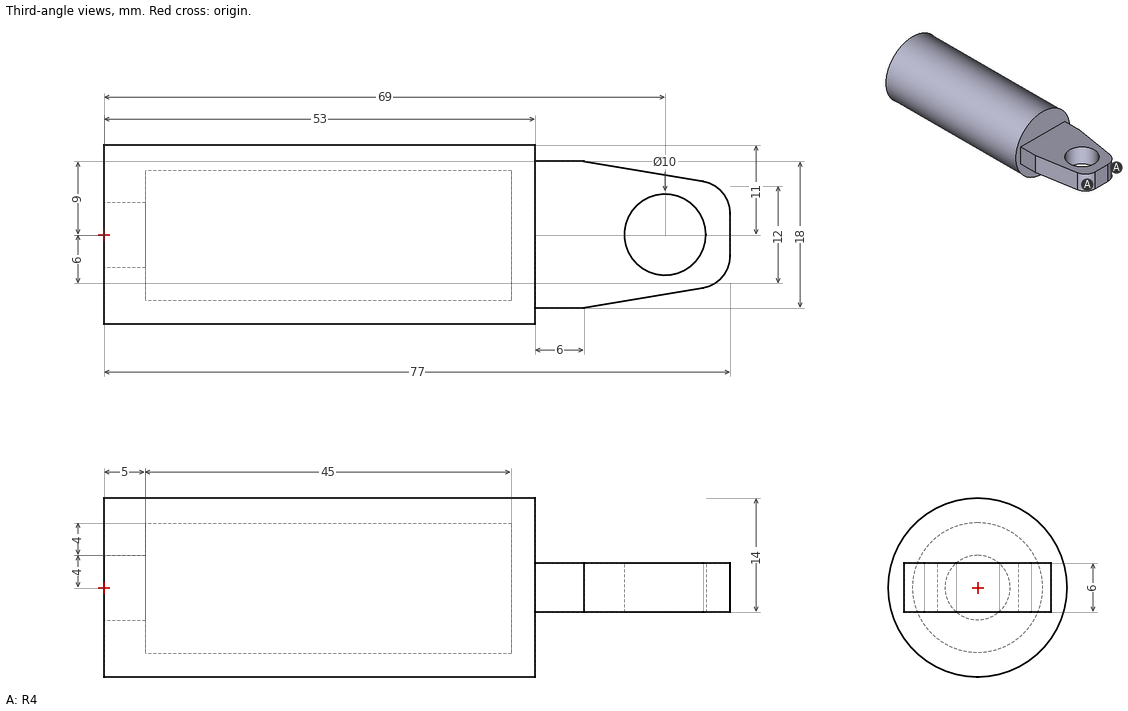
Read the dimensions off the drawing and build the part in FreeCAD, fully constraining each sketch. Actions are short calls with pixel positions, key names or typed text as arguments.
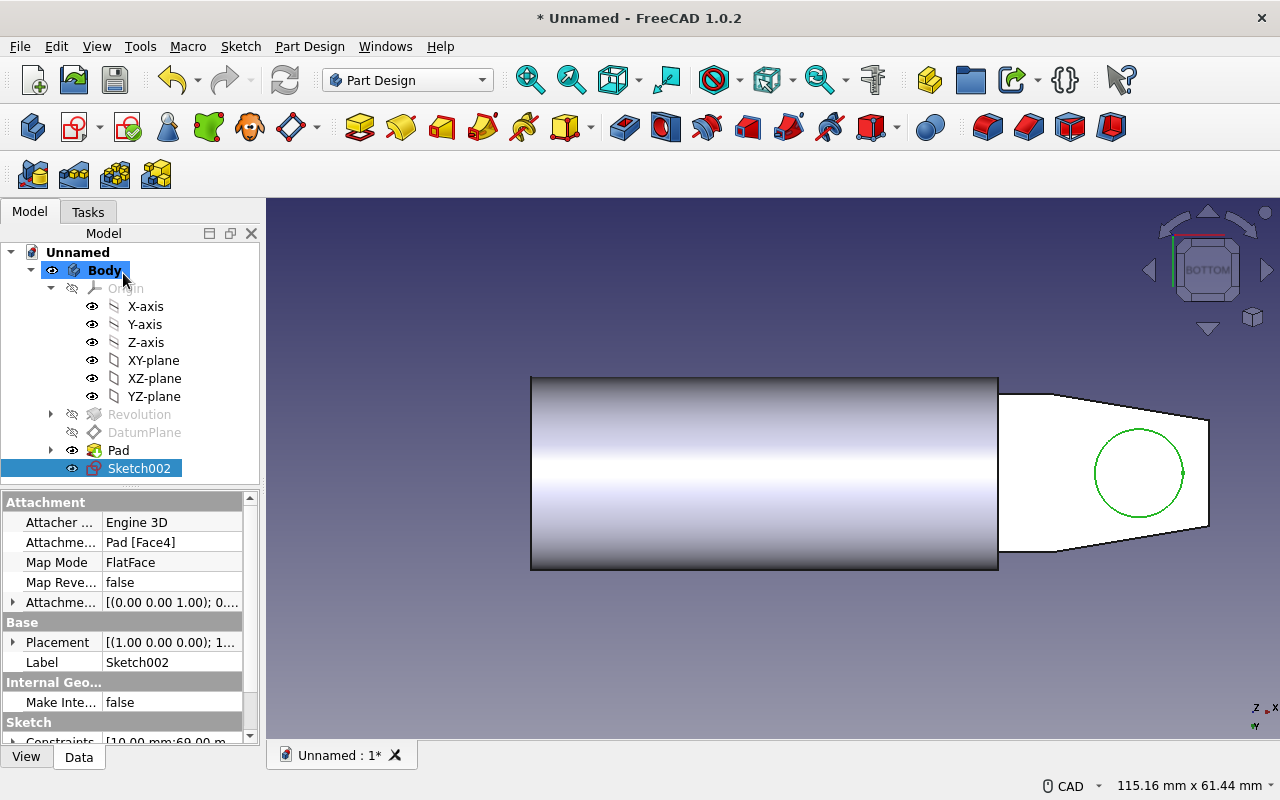
click(625, 128)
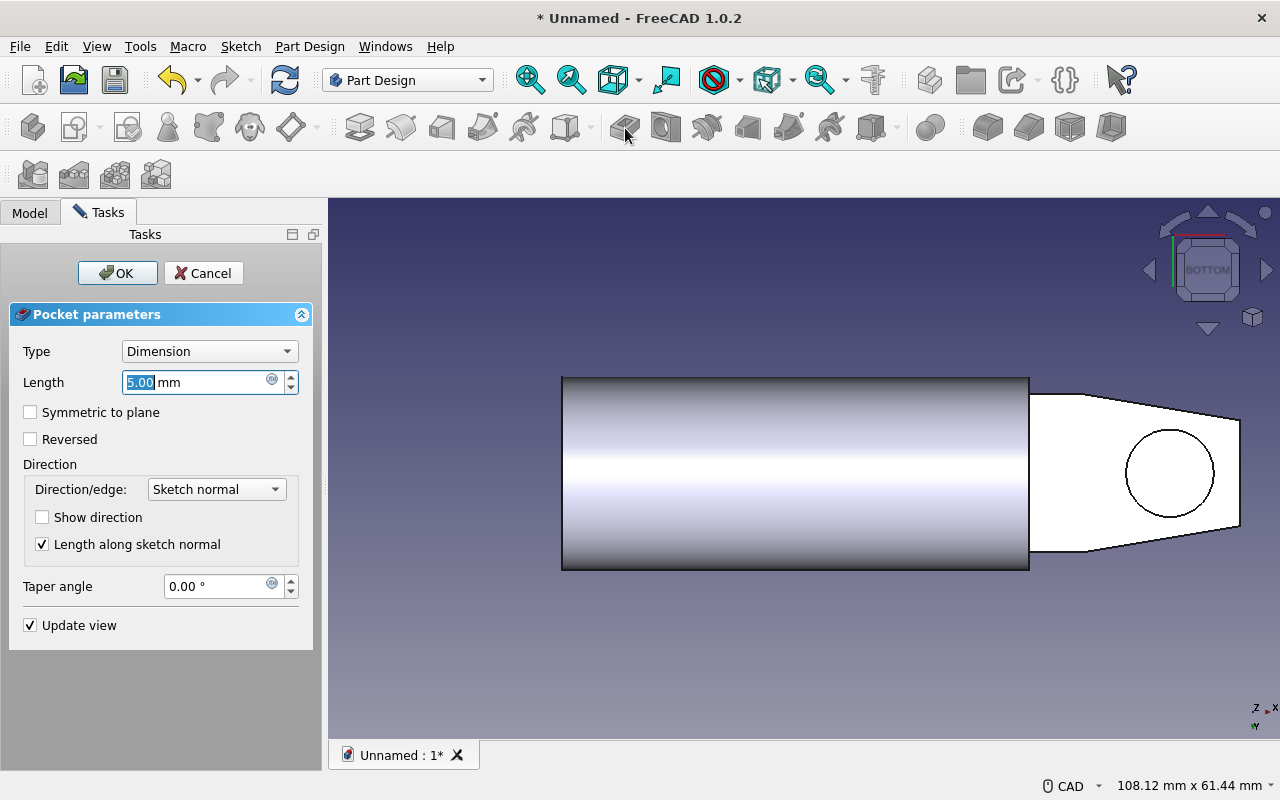
text(14)
key(Tab)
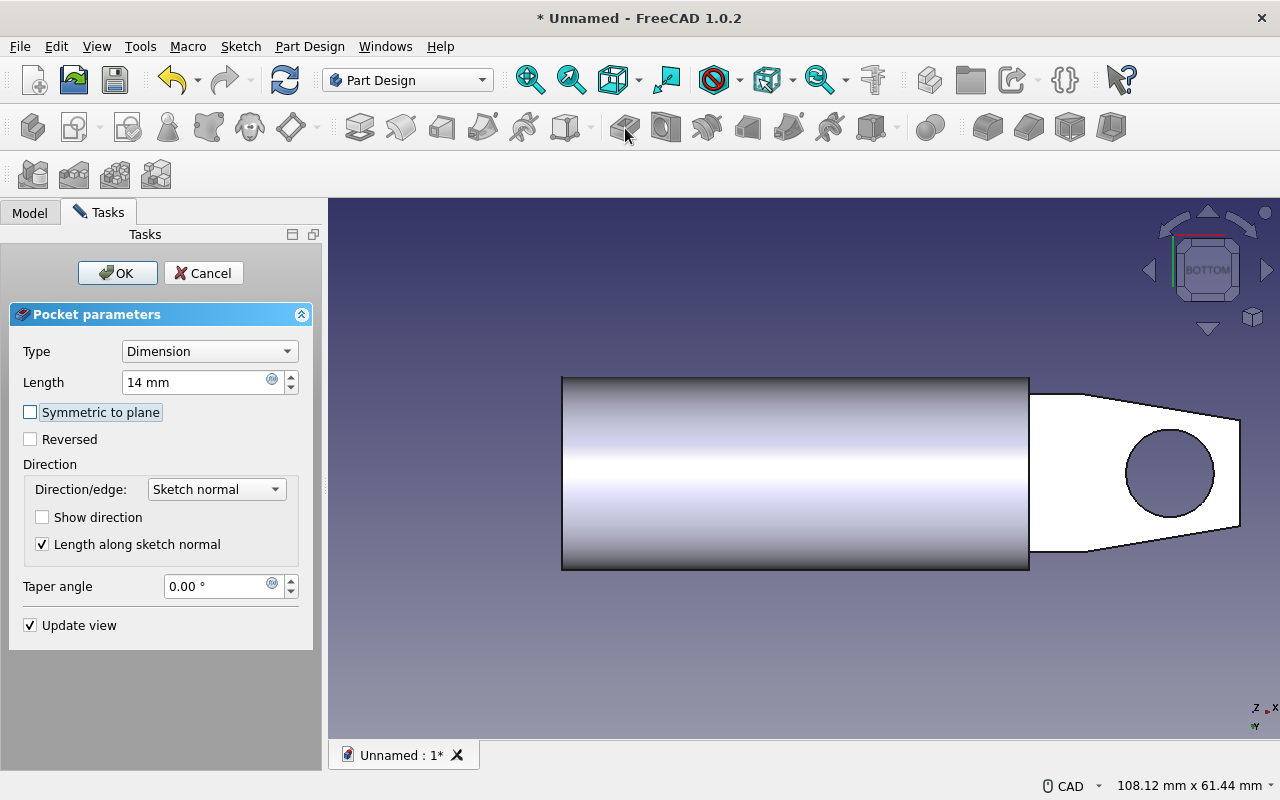
click(118, 273)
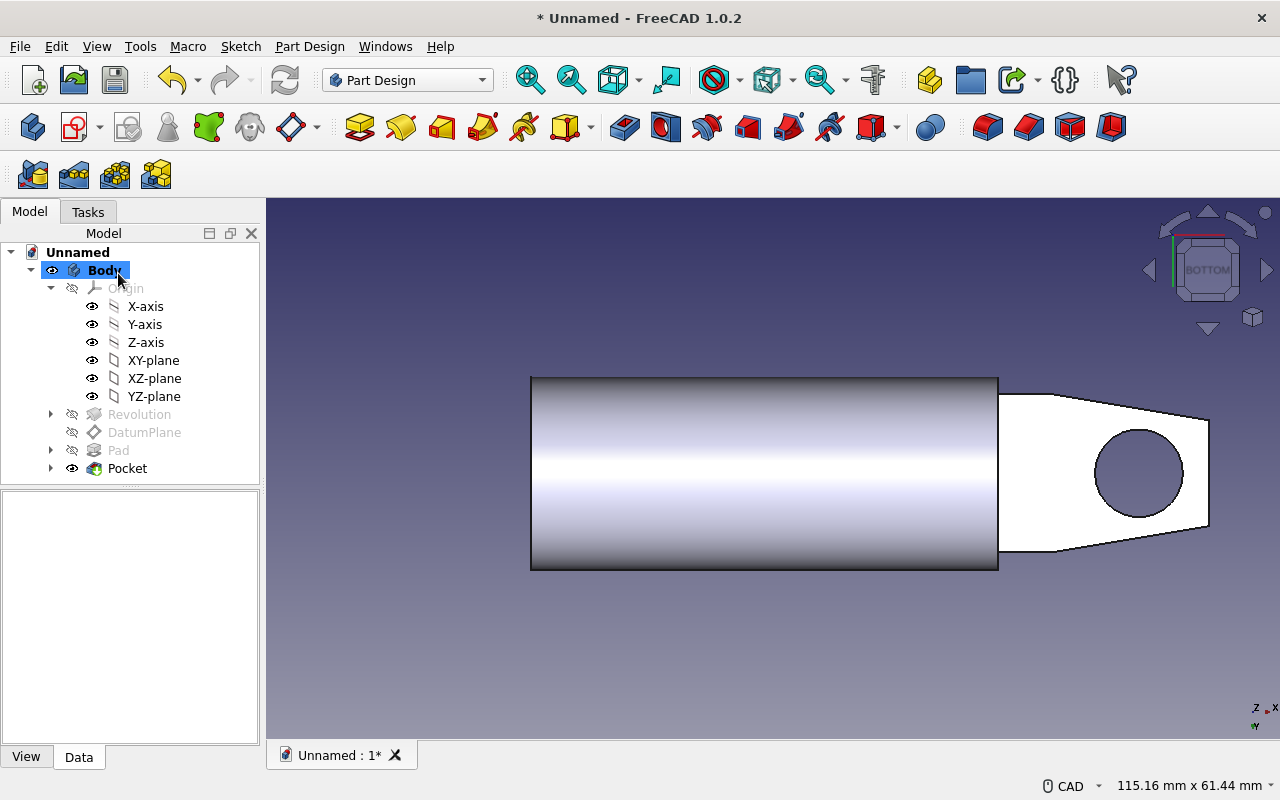
click(74, 128)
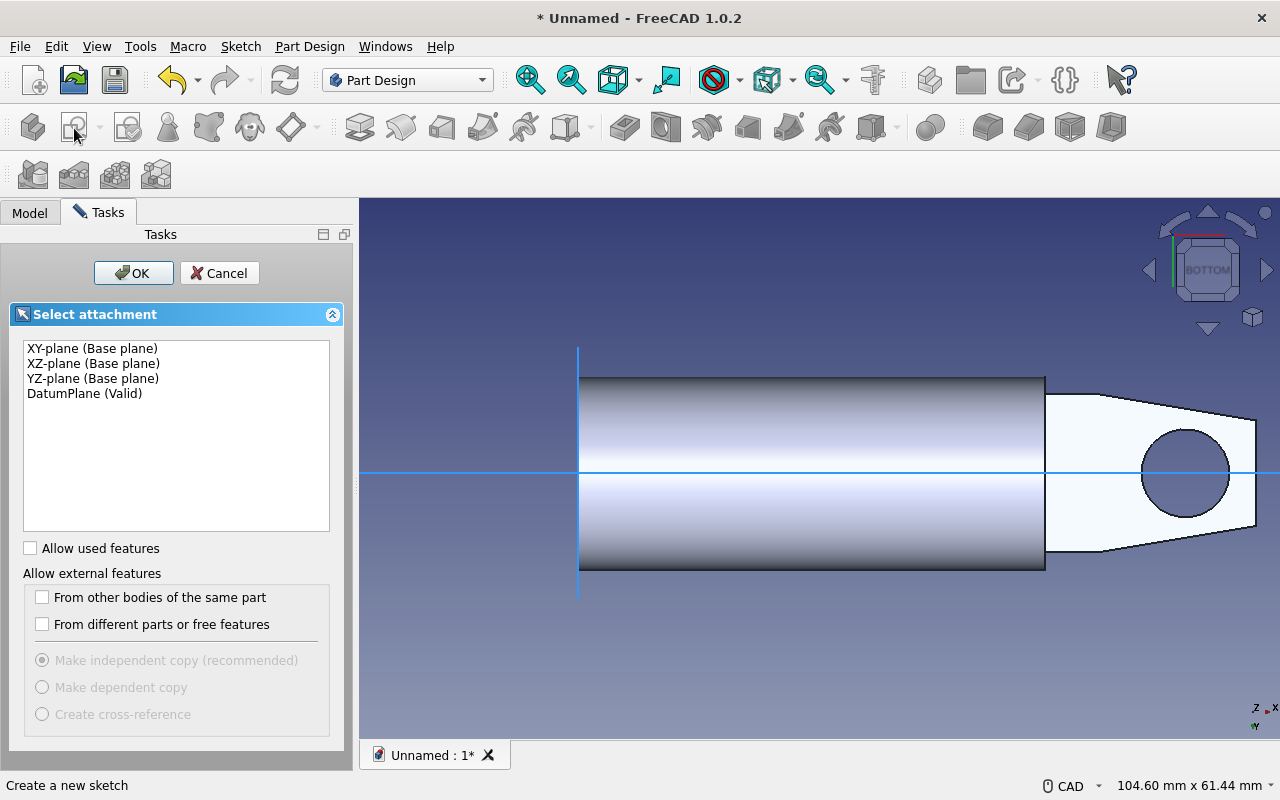
click(84, 364)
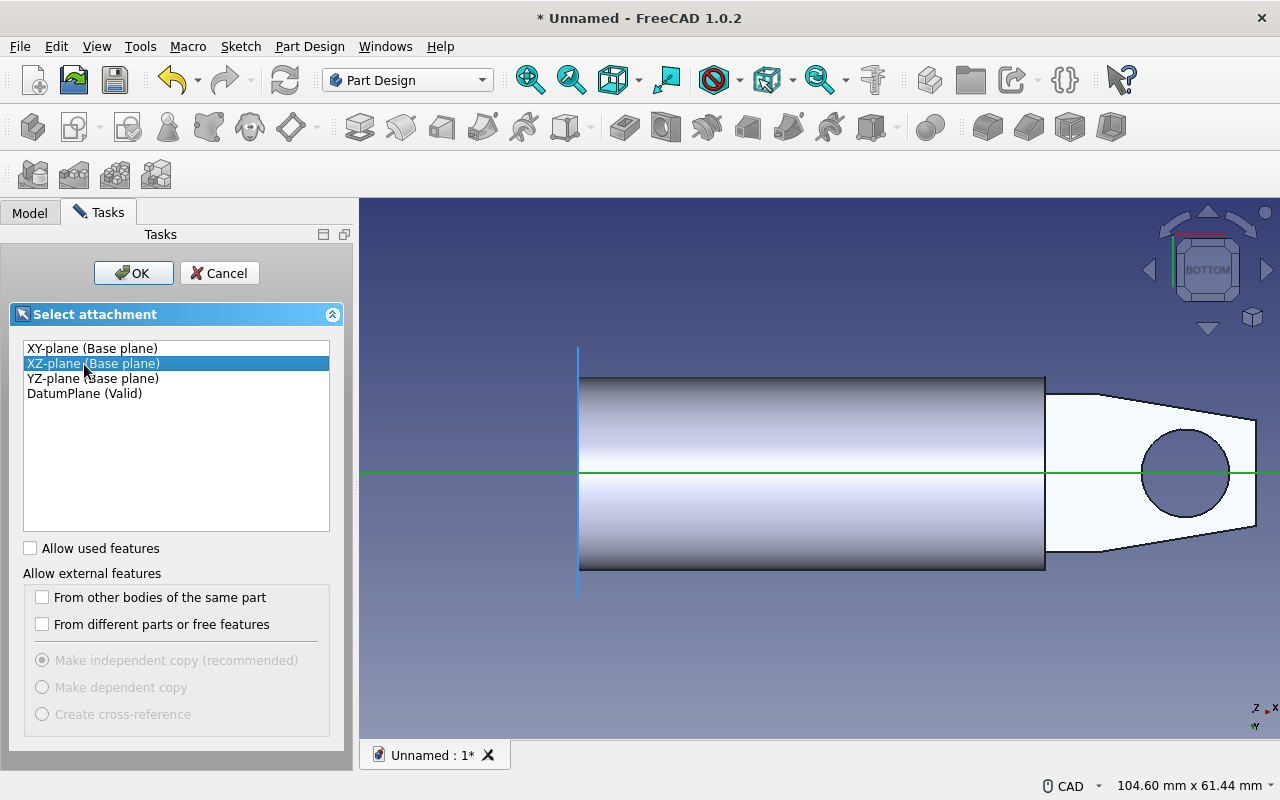
click(134, 273)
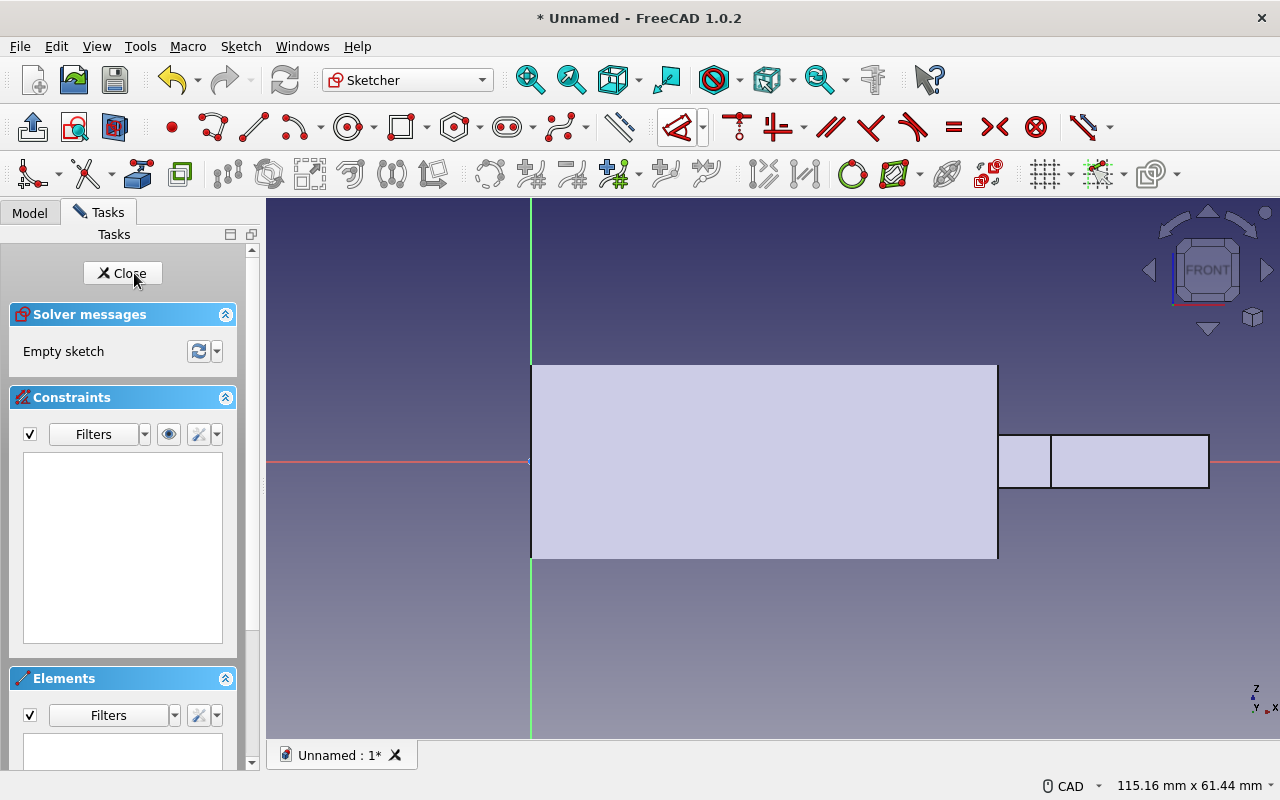
click(115, 128)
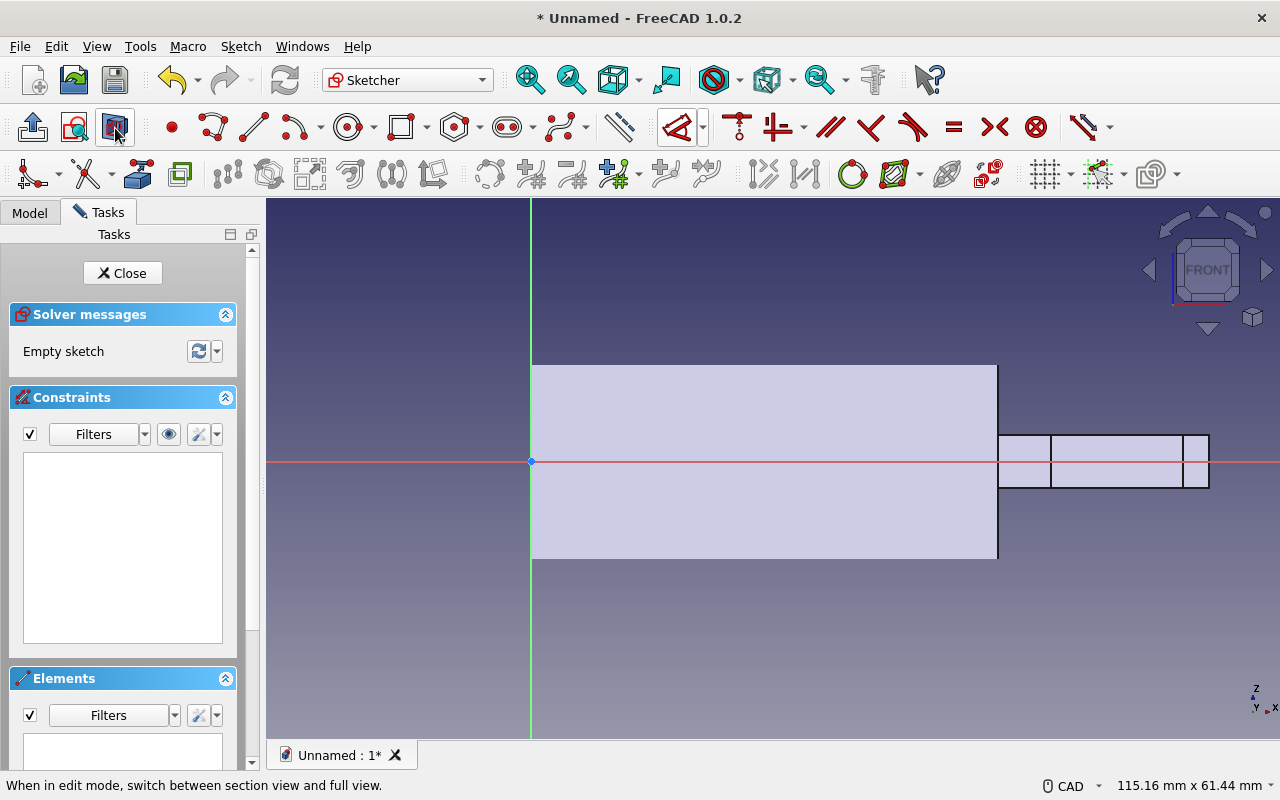
key(g)
key(m)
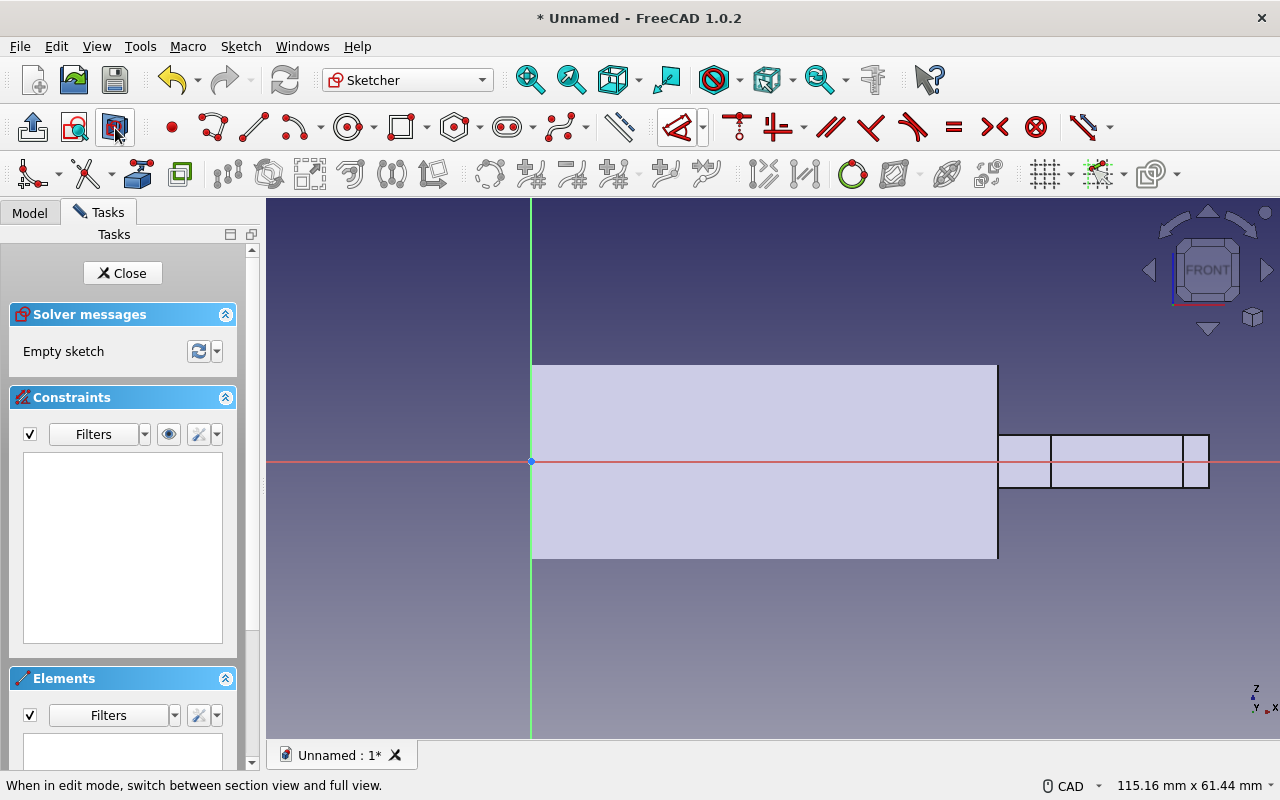
click(531, 462)
click(540, 427)
click(575, 427)
click(575, 391)
click(972, 391)
click(972, 453)
click(531, 462)
key(Escape)
key(Escape)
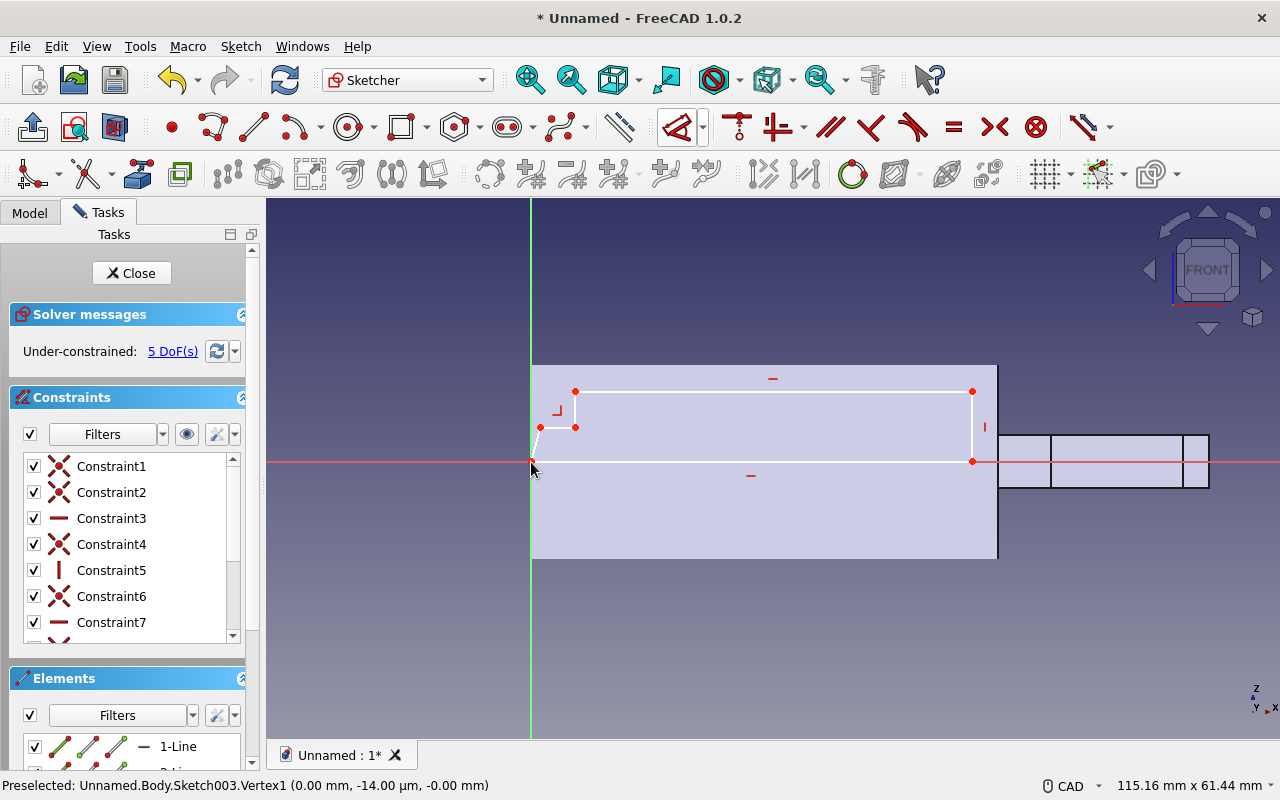
scroll(534, 452, up, 2)